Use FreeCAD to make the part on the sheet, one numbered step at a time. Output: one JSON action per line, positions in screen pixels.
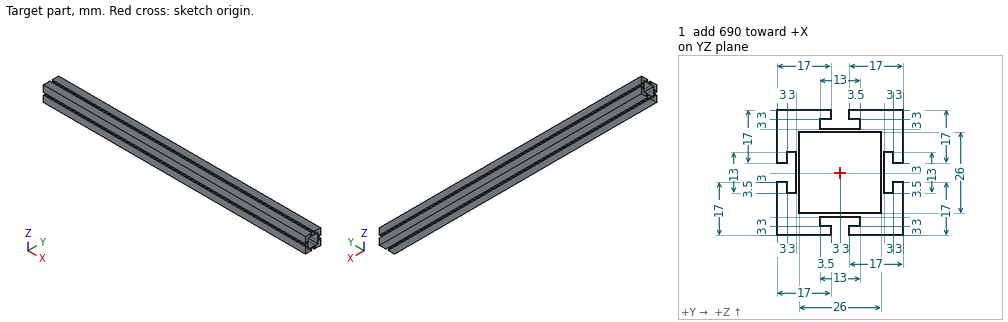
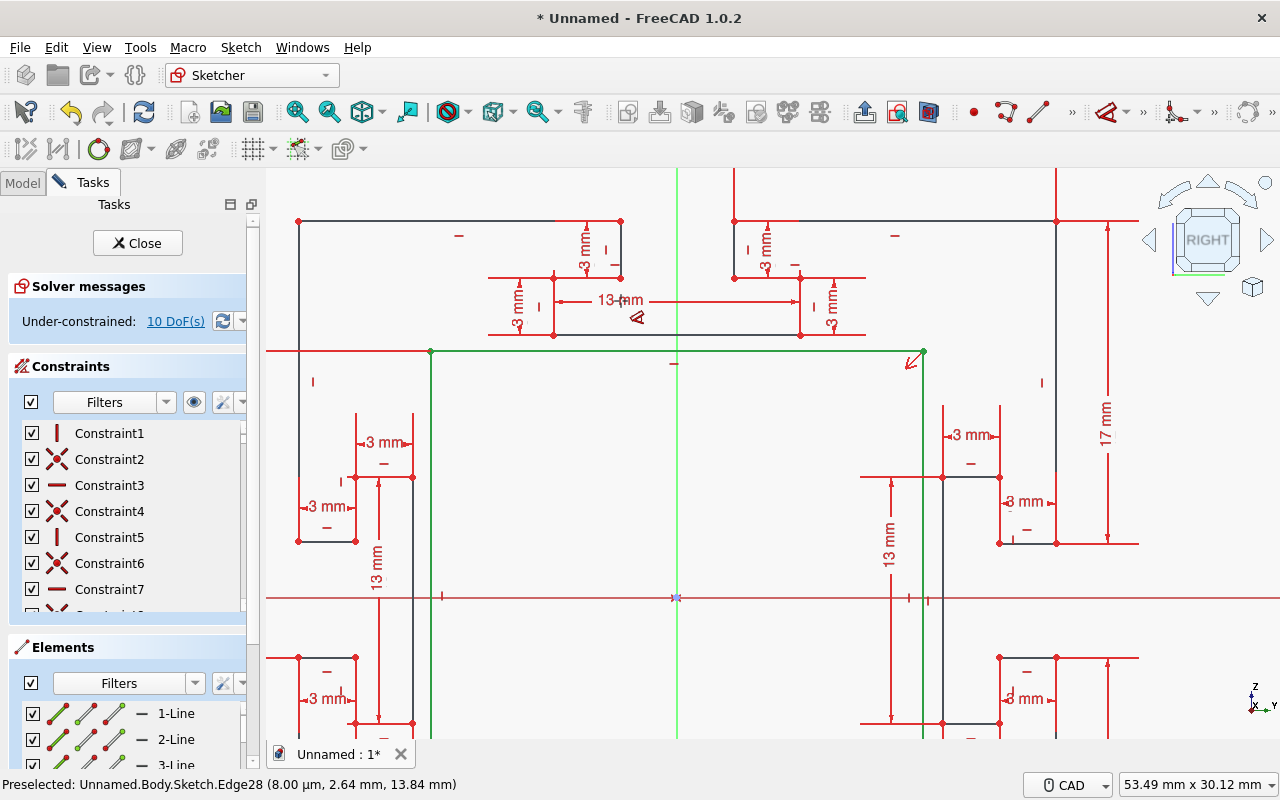
{"action": "left_click", "coordinate": [524, 221]}
{"action": "left_click", "coordinate": [460, 255]}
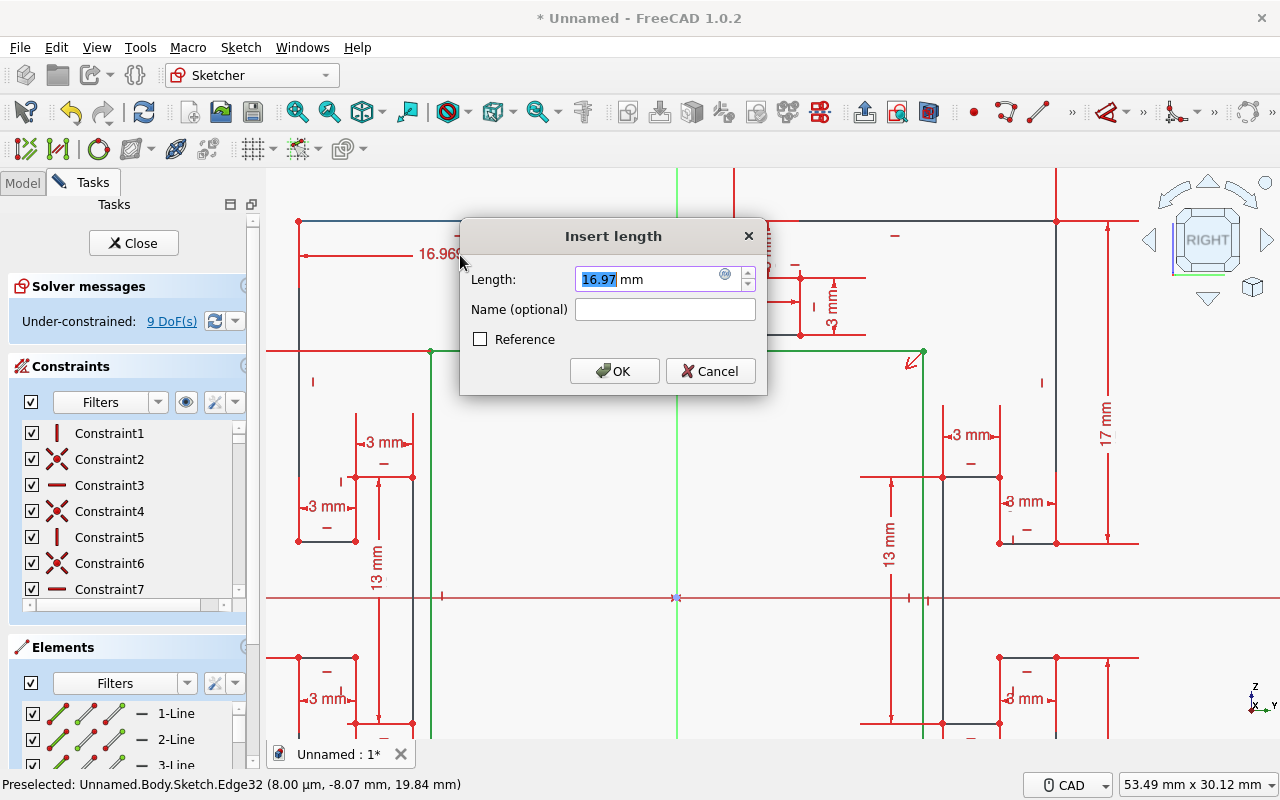
{"action": "type", "text": "17"}
{"action": "key", "text": "Return"}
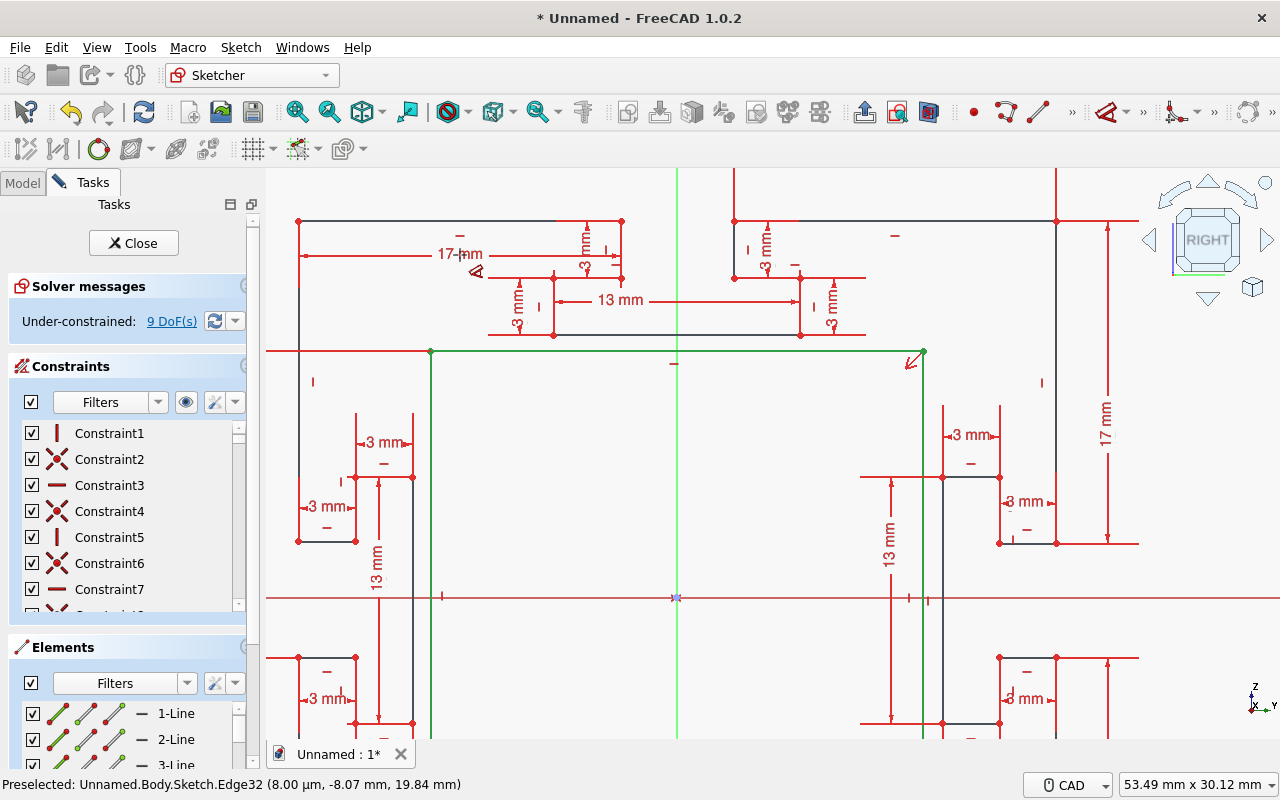
{"action": "left_click", "coordinate": [299, 318]}
{"action": "left_click", "coordinate": [333, 382]}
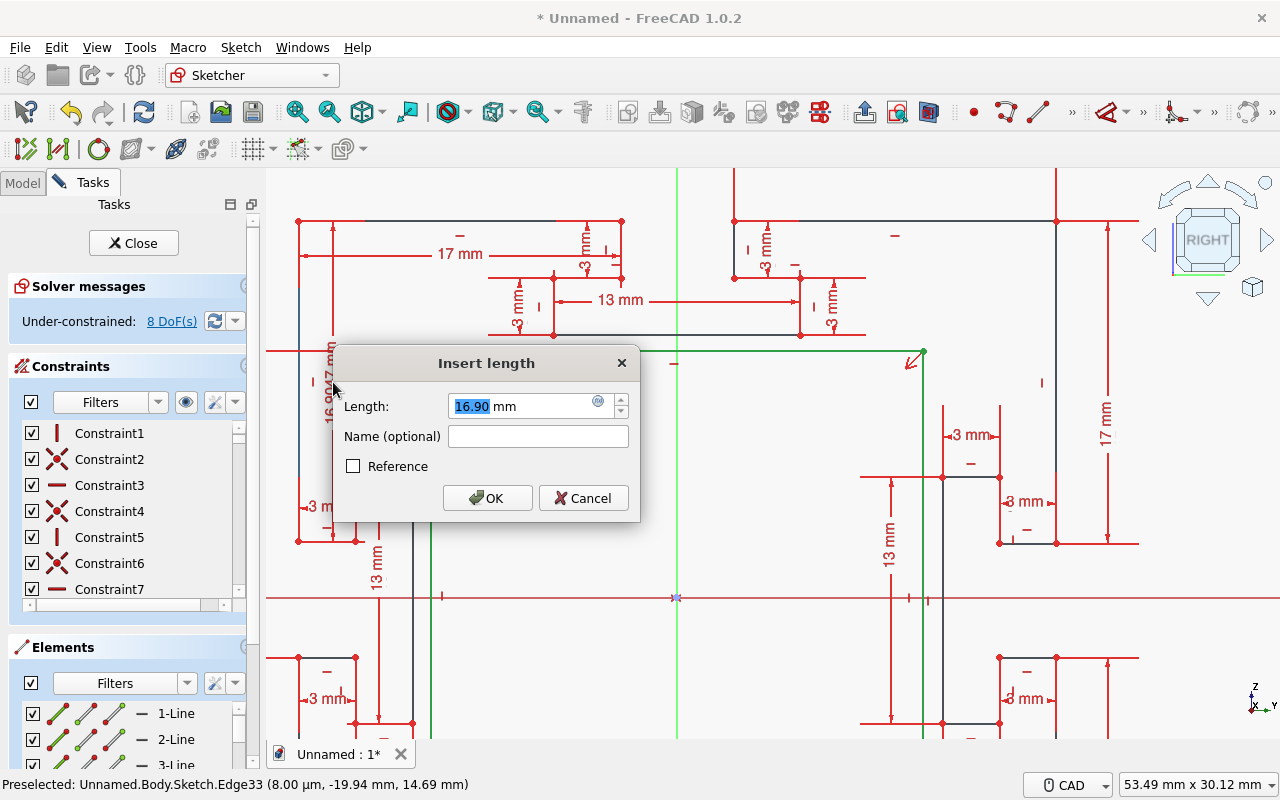
{"action": "type", "text": "17"}
{"action": "key", "text": "Return"}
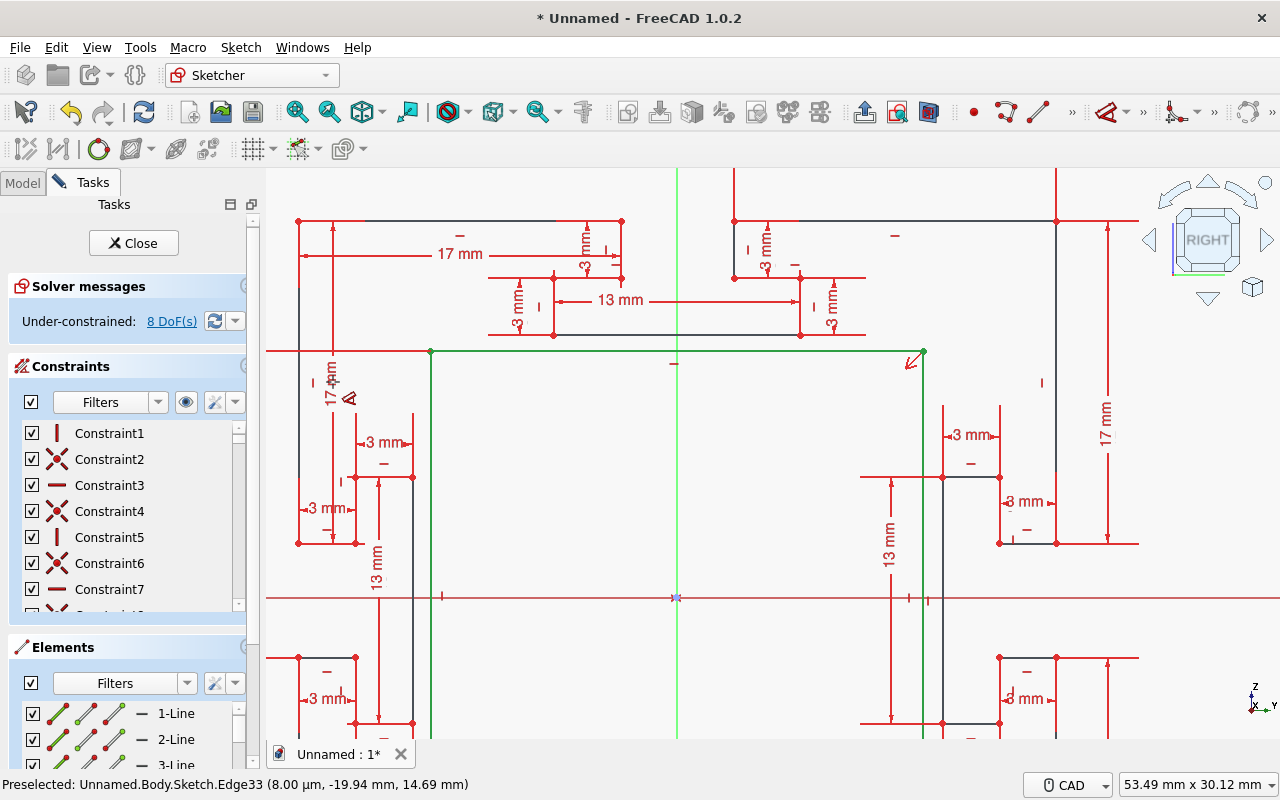
{"action": "left_click", "coordinate": [356, 658]}
{"action": "left_click", "coordinate": [322, 628]}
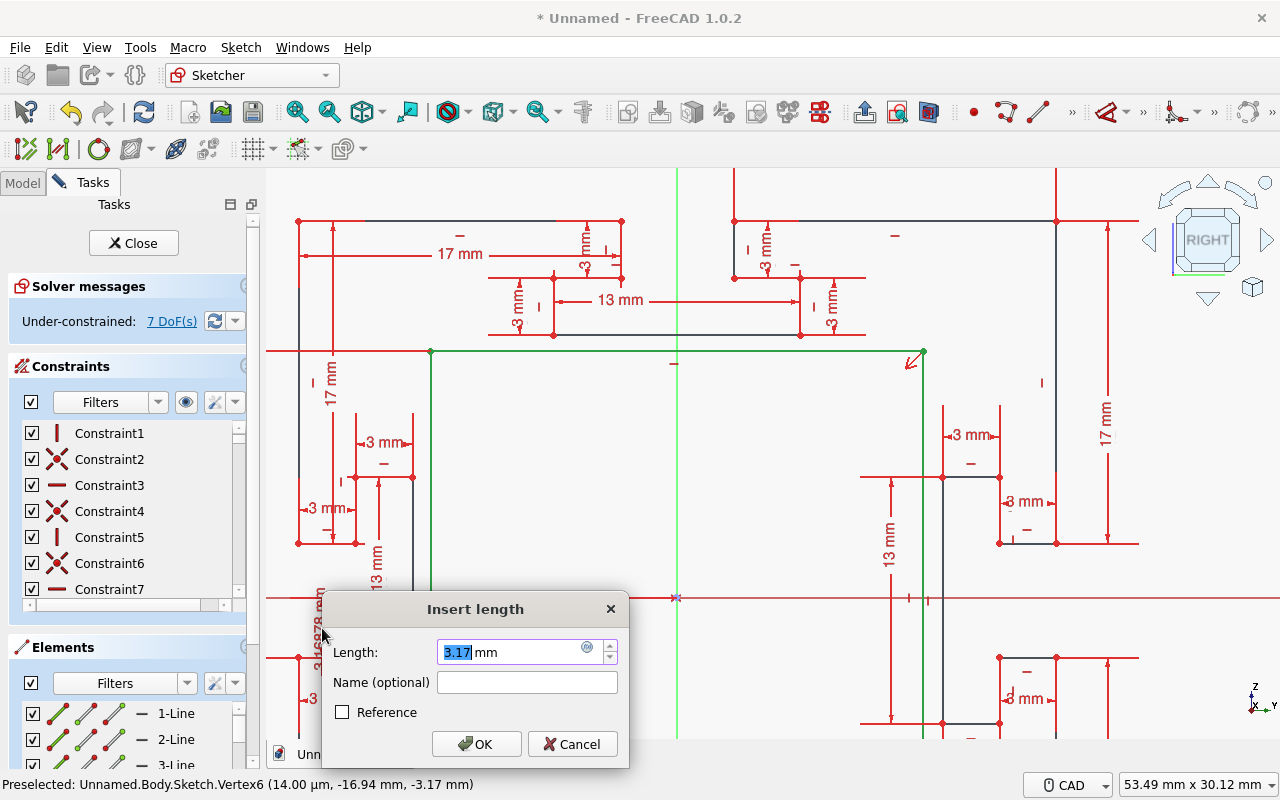
{"action": "type", "text": "3"}
{"action": "key", "text": "Return"}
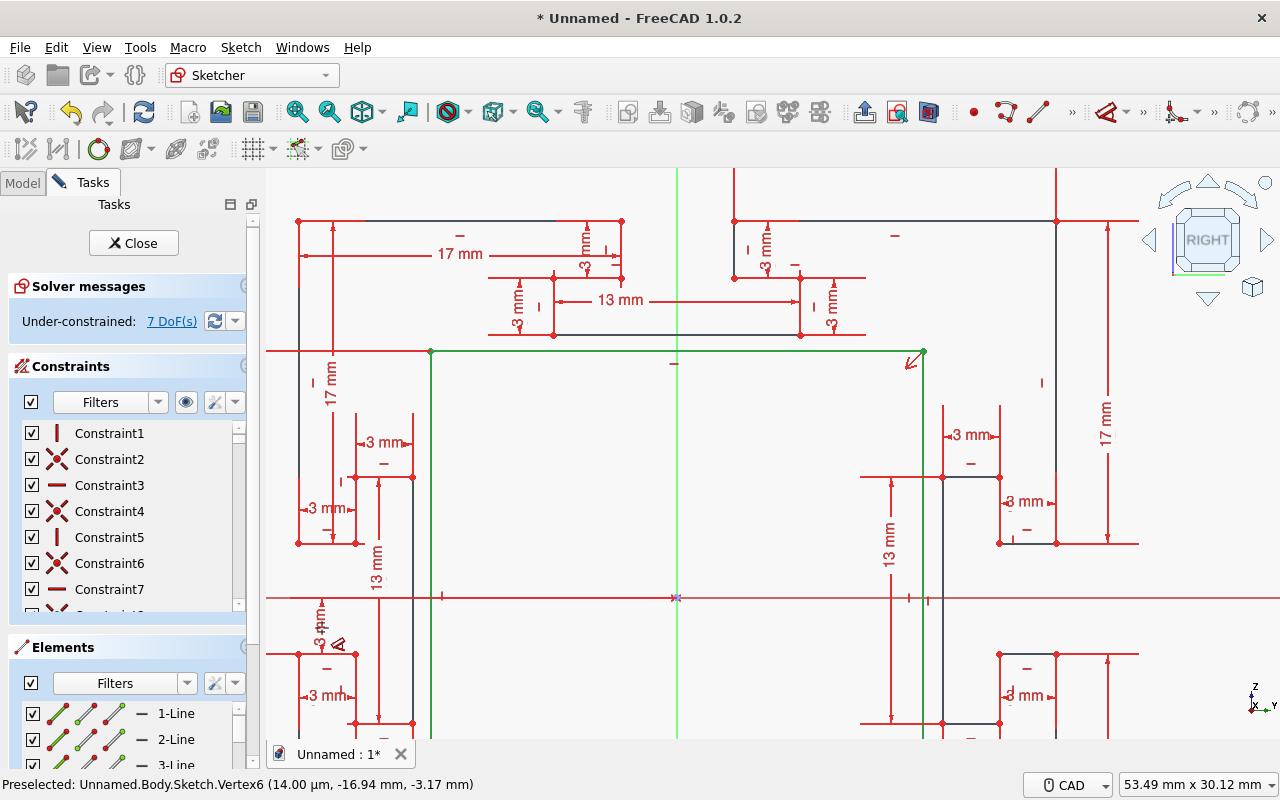
{"action": "scroll", "coordinate": [727, 336], "scroll_direction": "down", "scroll_amount": 4}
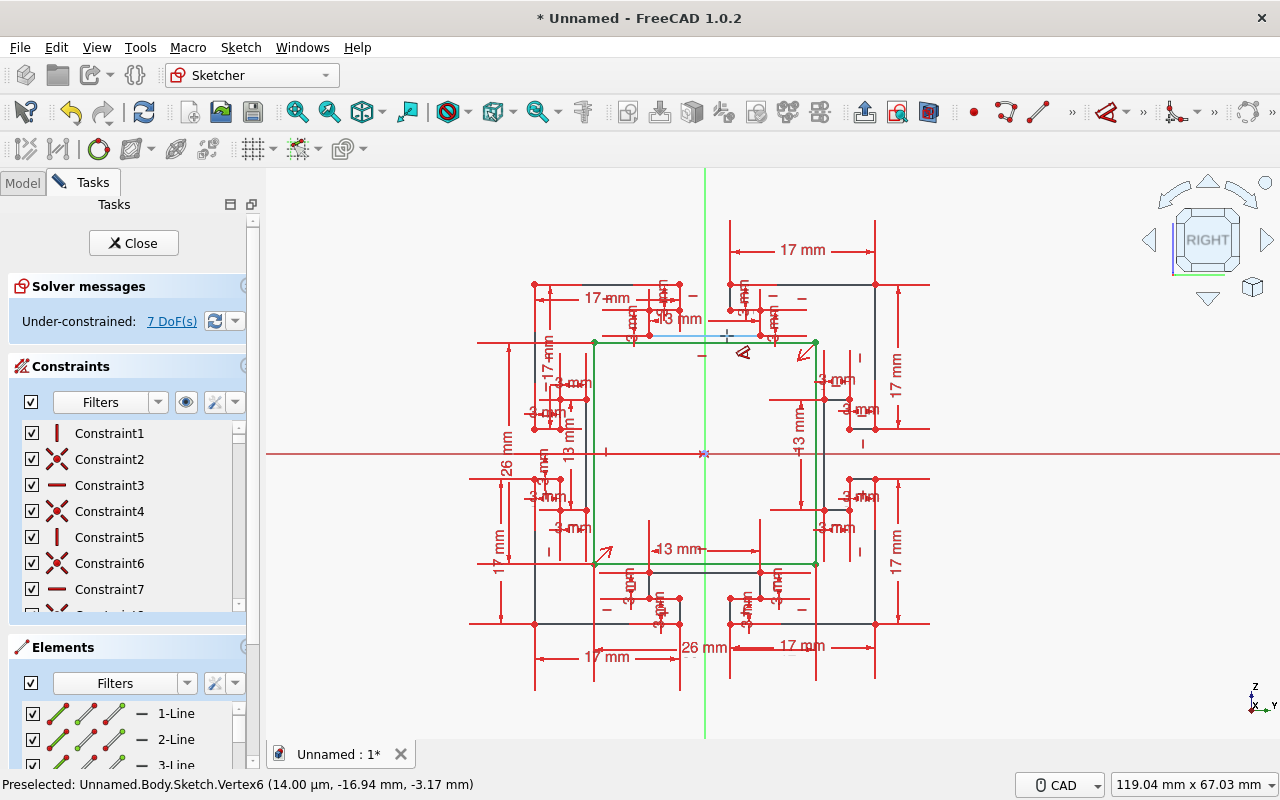
{"action": "scroll", "coordinate": [680, 624], "scroll_direction": "up", "scroll_amount": 3}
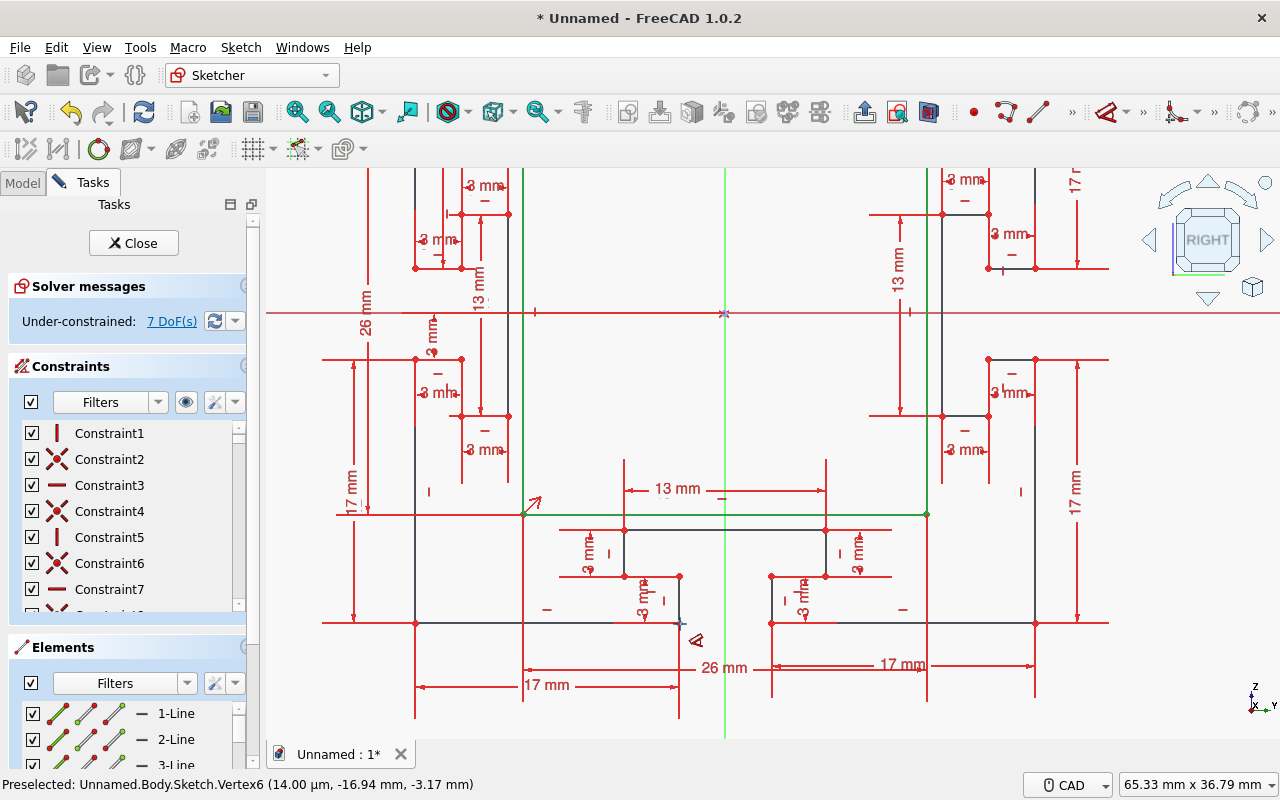
{"action": "left_click", "coordinate": [679, 623]}
{"action": "left_click", "coordinate": [702, 657]}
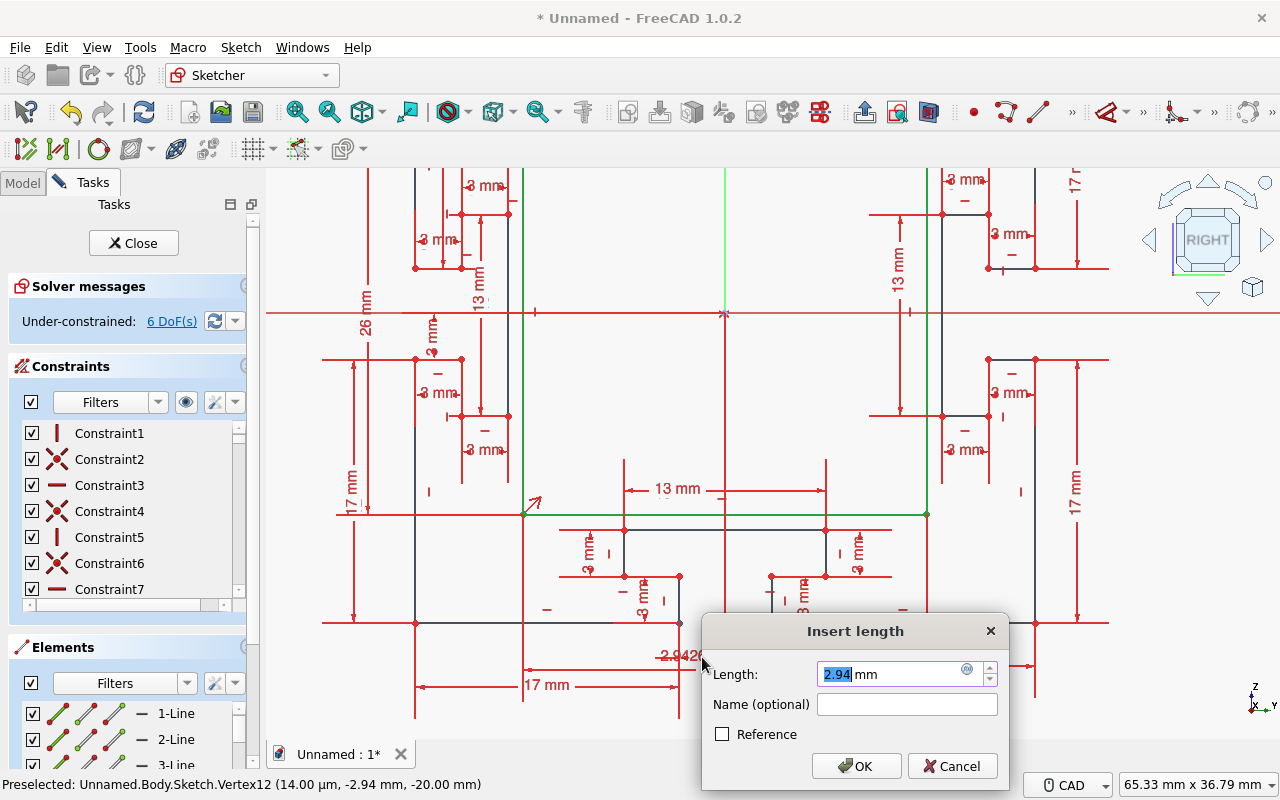
{"action": "type", "text": "3"}
{"action": "key", "text": "Return"}